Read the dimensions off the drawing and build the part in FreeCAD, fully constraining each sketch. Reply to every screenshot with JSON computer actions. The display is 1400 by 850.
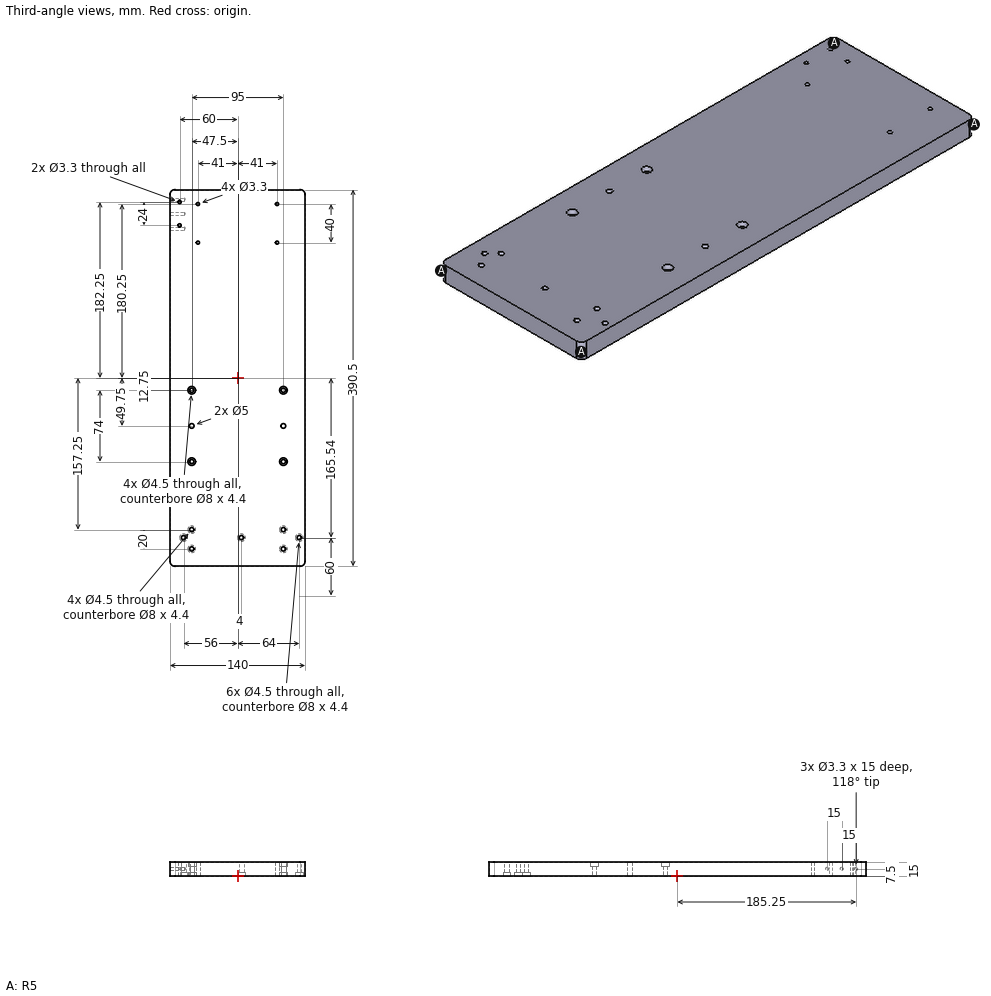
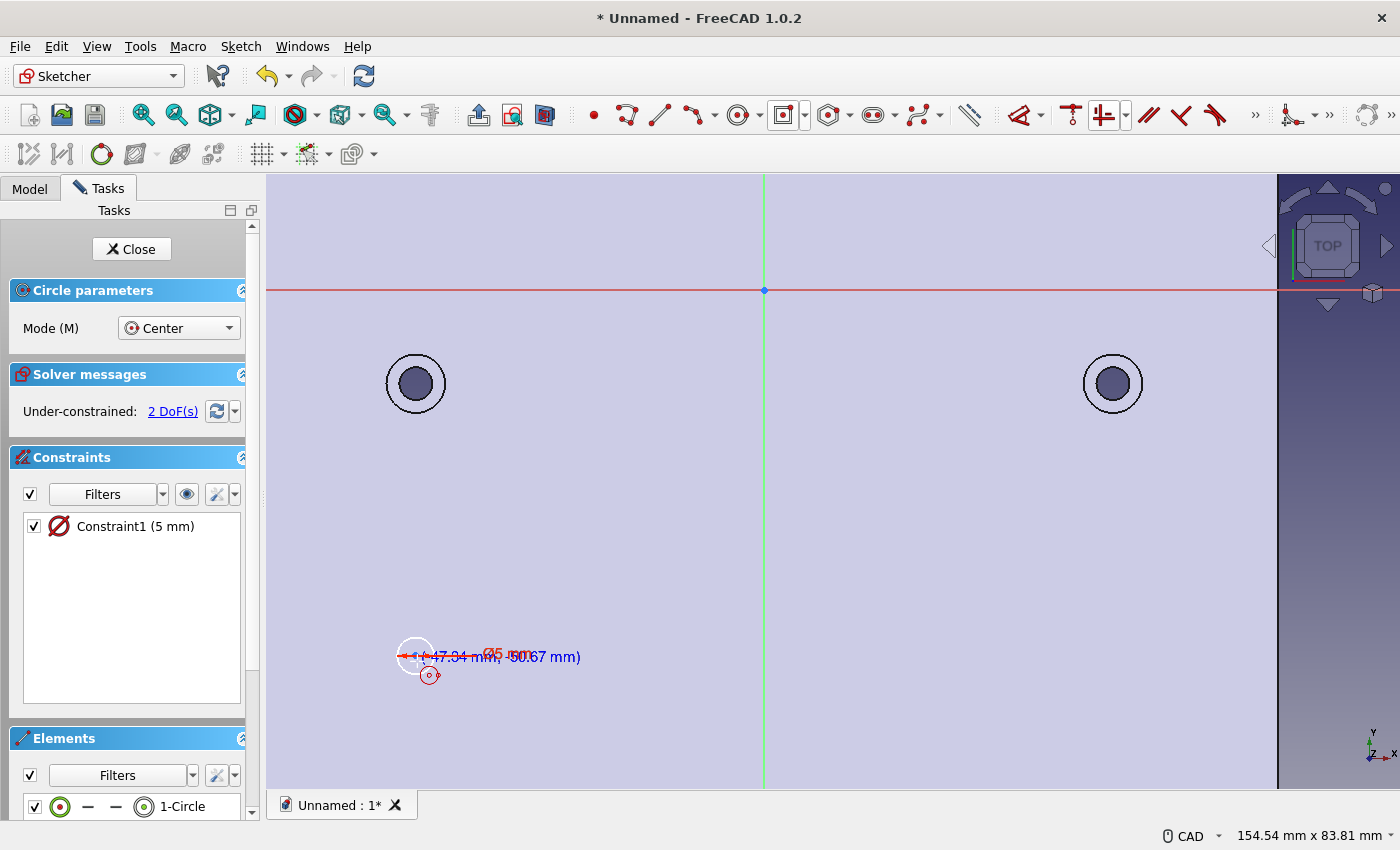
{"action": "scroll", "coordinate": [1113, 655], "scroll_direction": "up", "scroll_amount": 2}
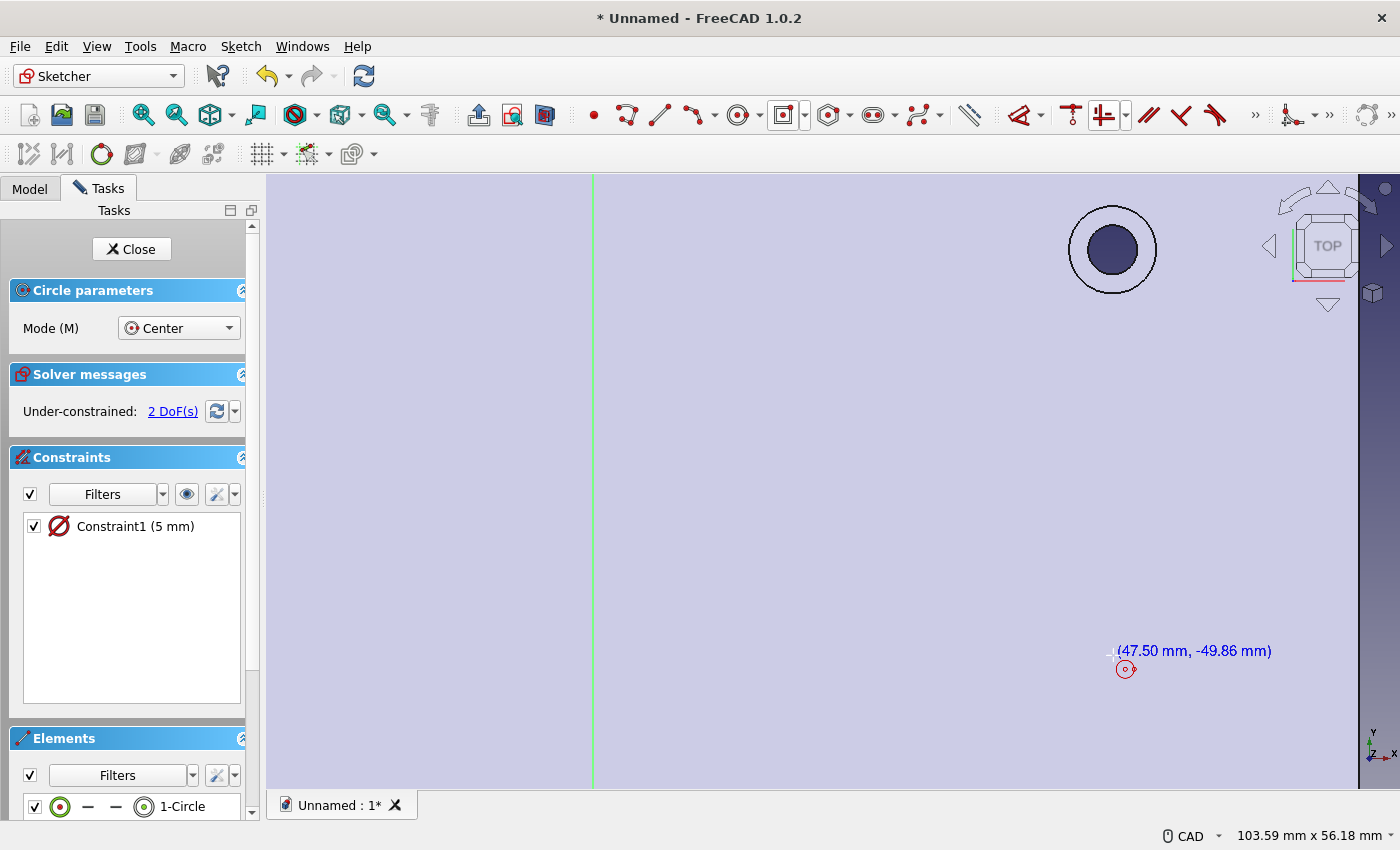
{"action": "left_click", "coordinate": [1113, 655]}
{"action": "mouse_move", "coordinate": [1132, 636]}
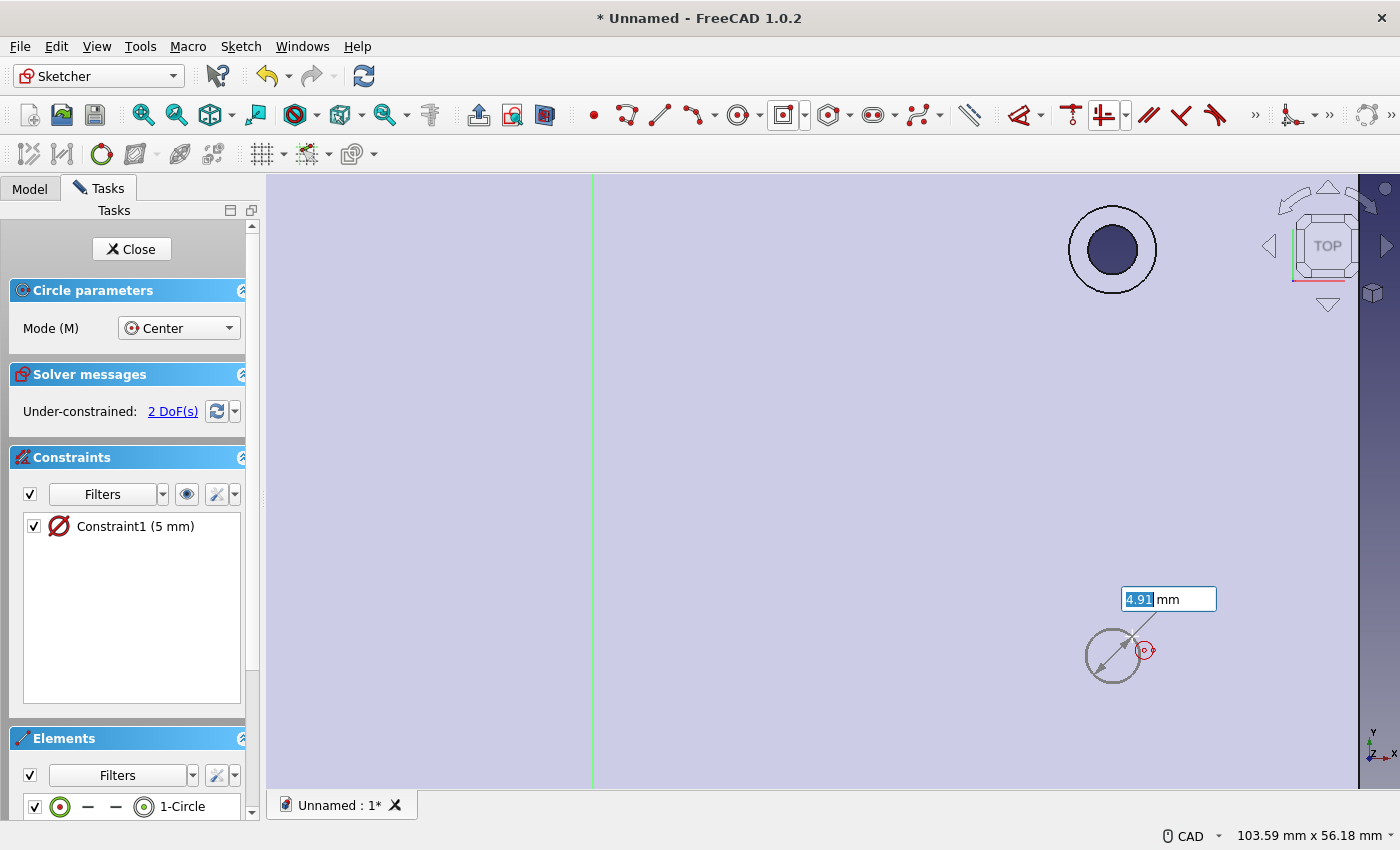
{"action": "type", "text": "5"}
{"action": "key", "text": "Return"}
{"action": "key", "text": "Escape"}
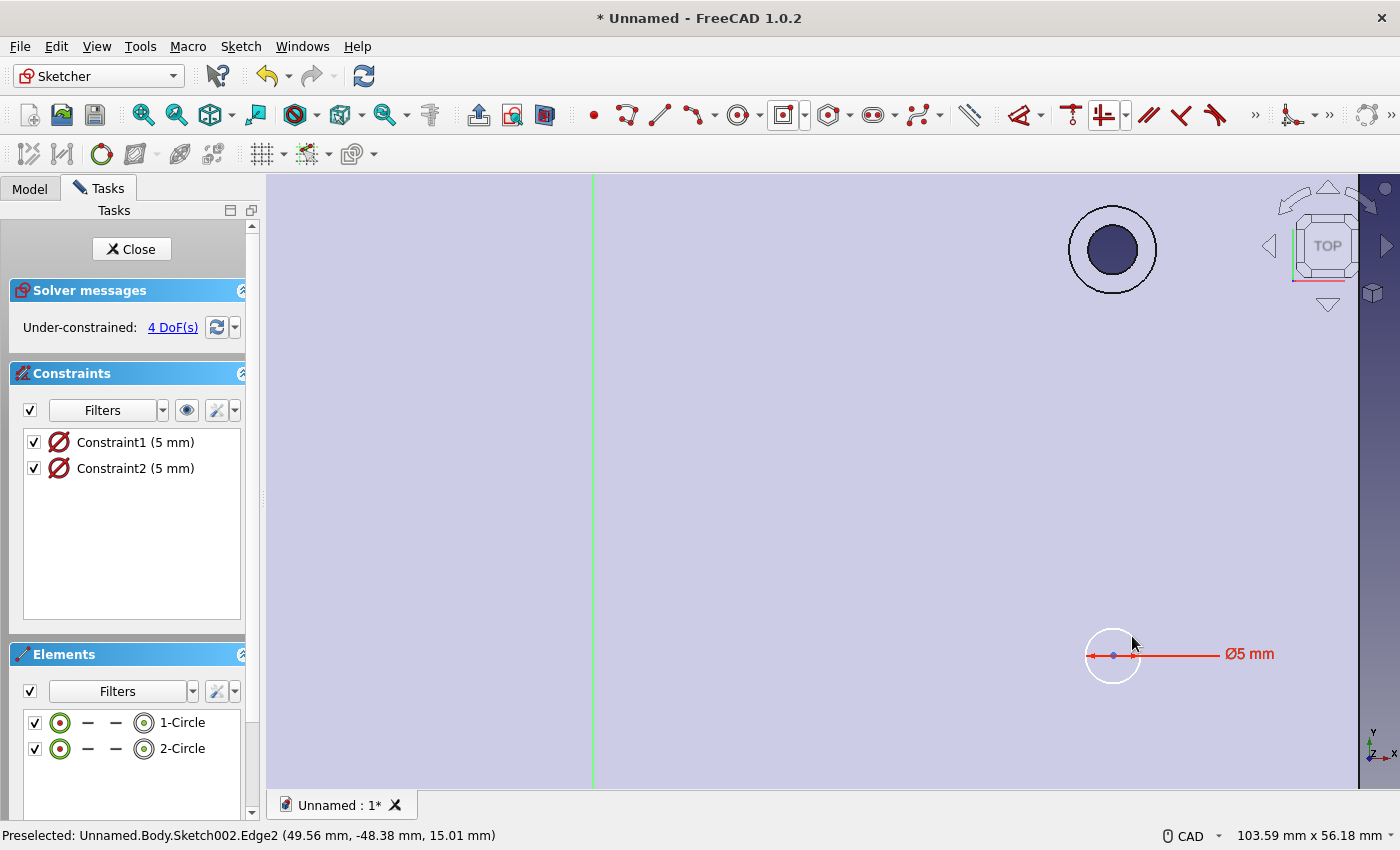
{"action": "scroll", "coordinate": [1114, 655], "scroll_direction": "down", "scroll_amount": 2}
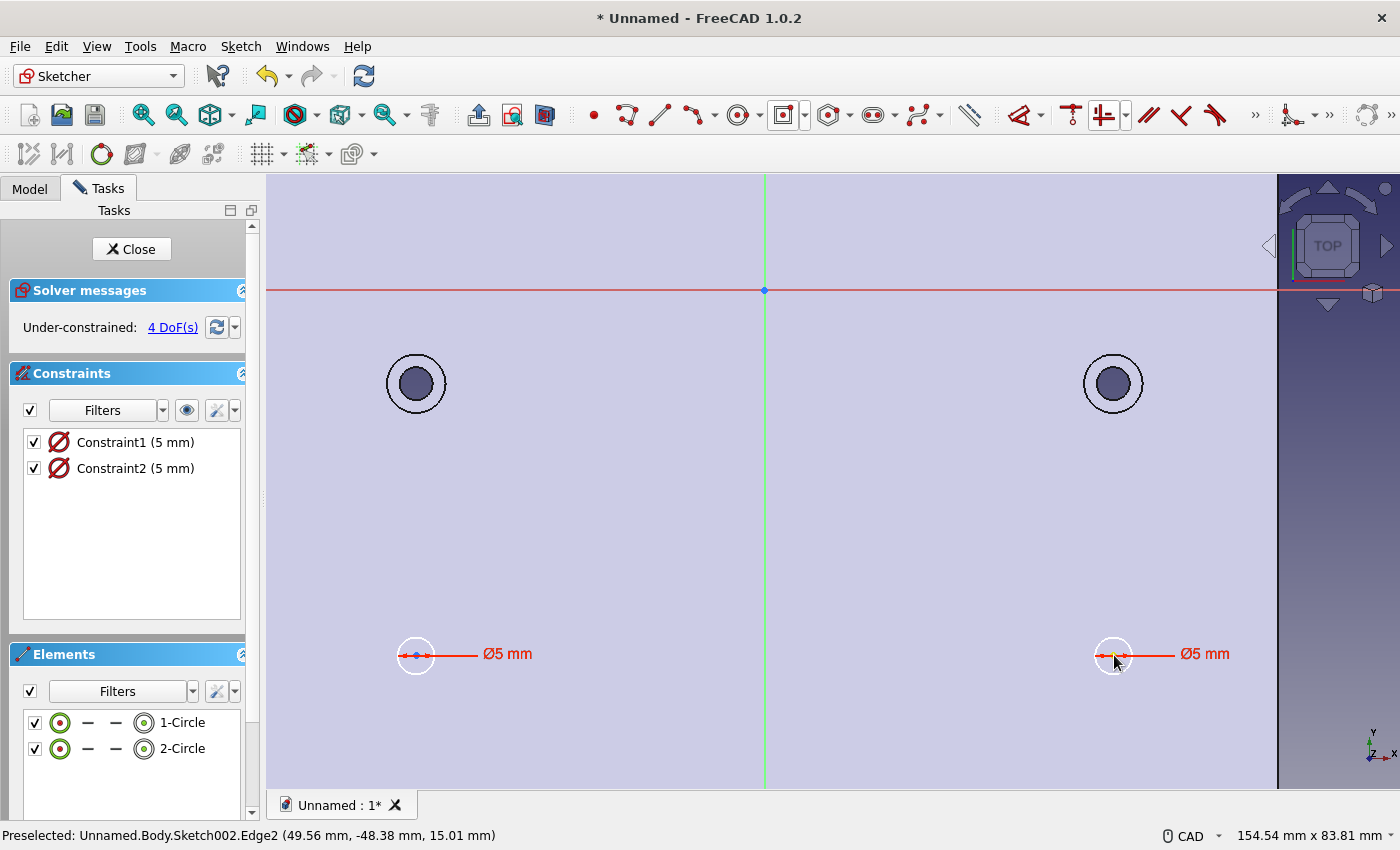
{"action": "left_click", "coordinate": [416, 656]}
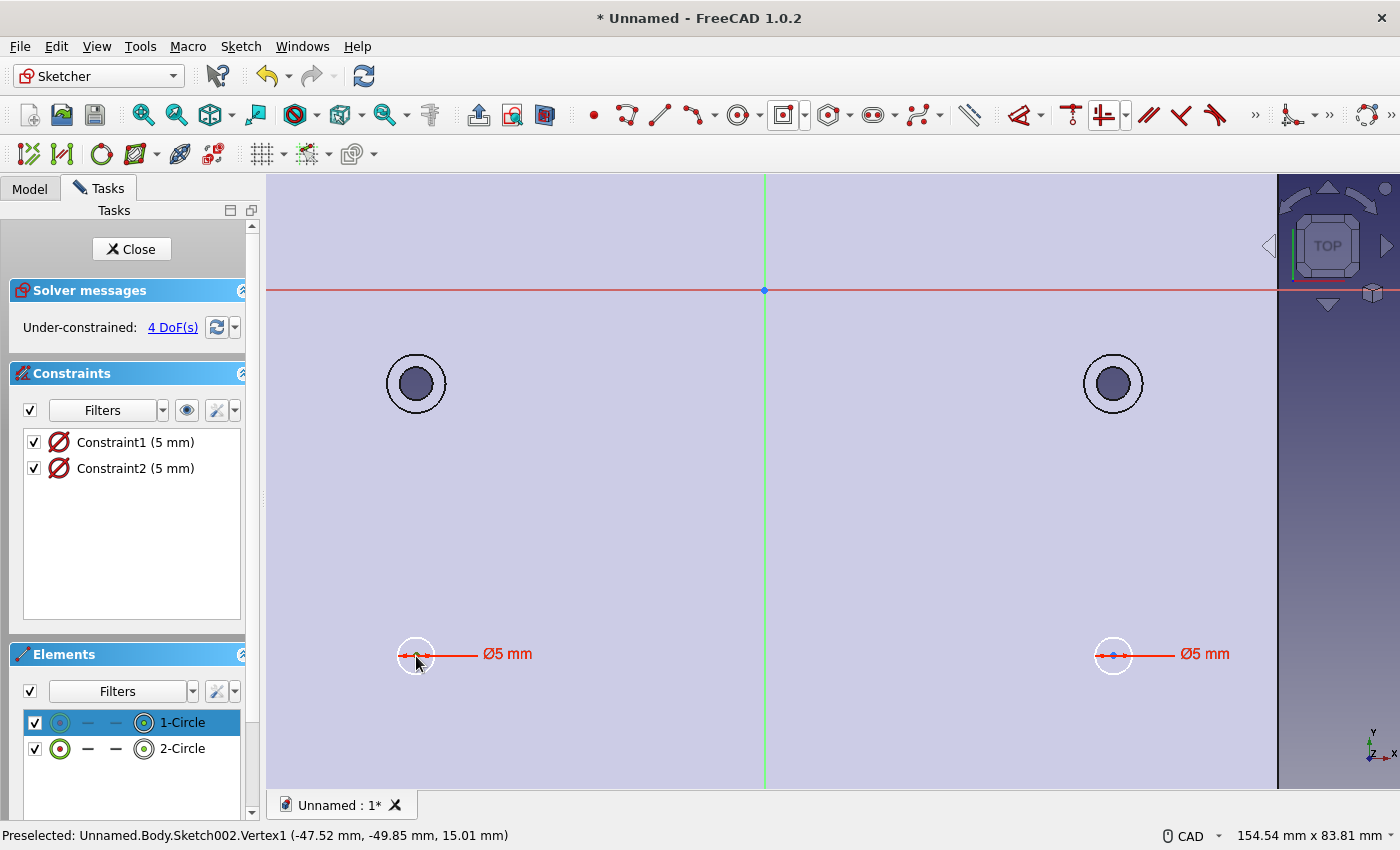
{"action": "left_click", "coordinate": [1114, 656]}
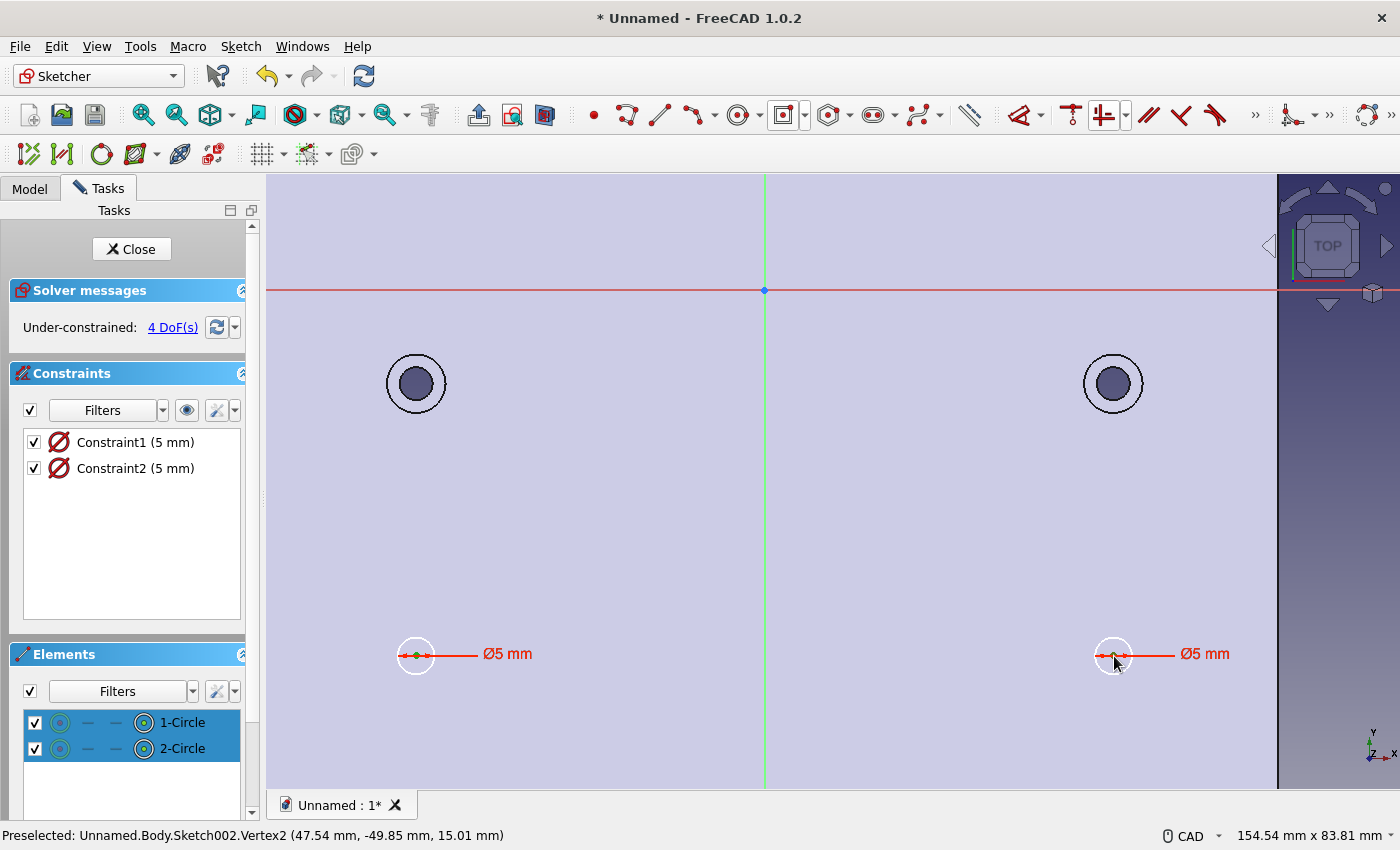
{"action": "key", "text": "h"}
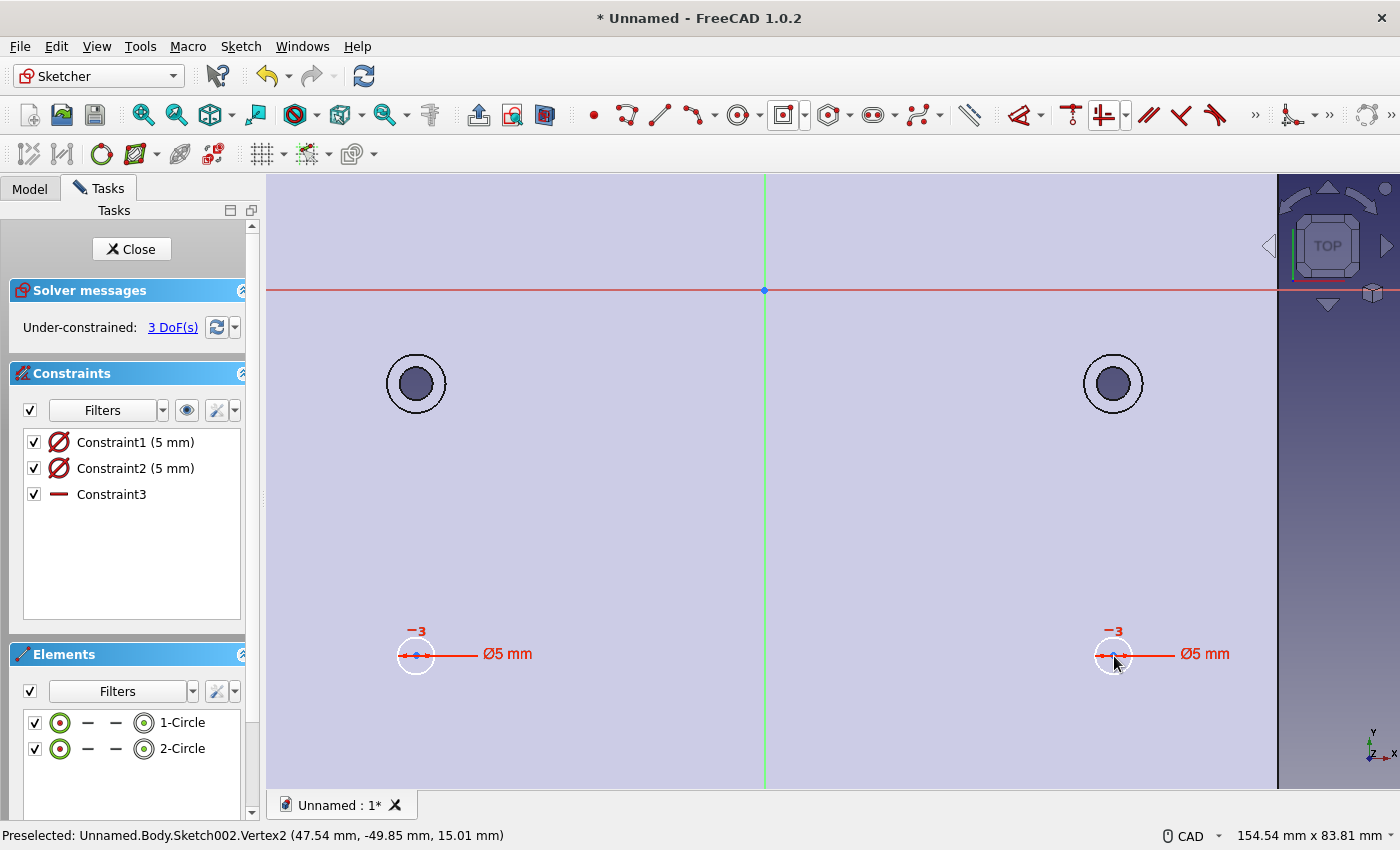
{"action": "left_click", "coordinate": [1018, 116]}